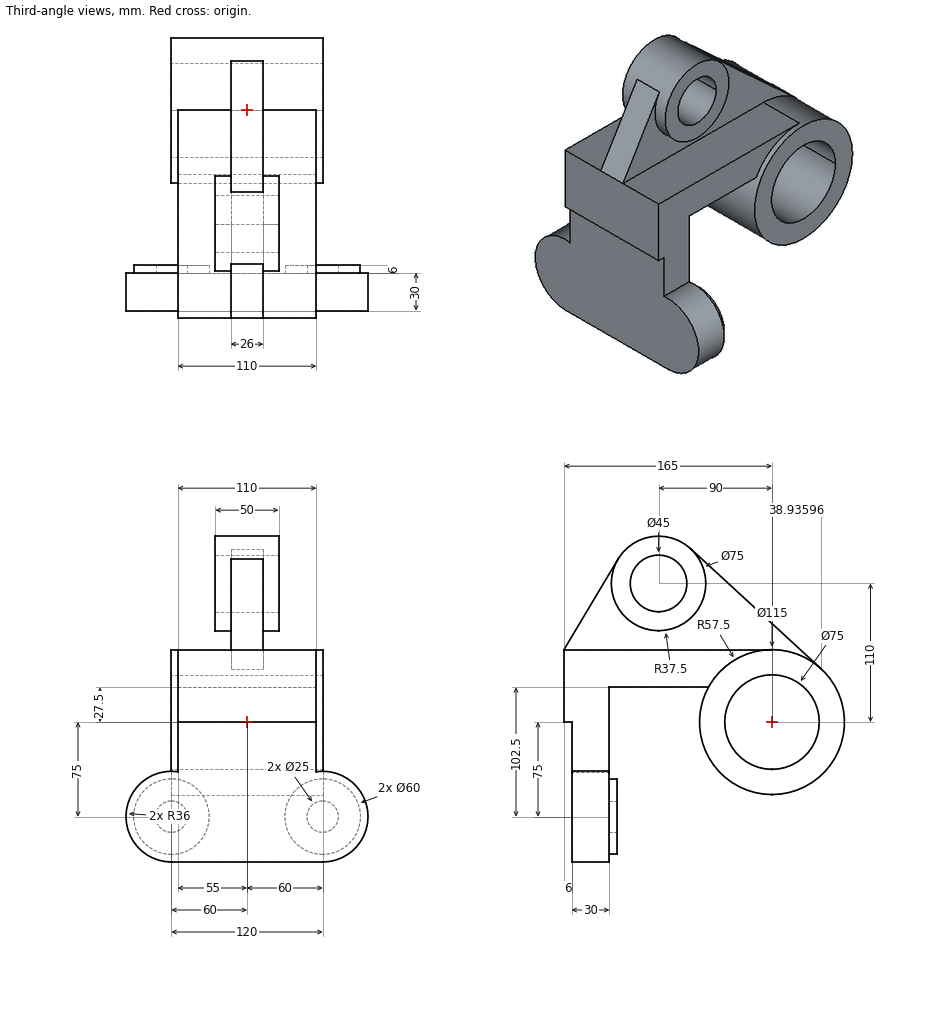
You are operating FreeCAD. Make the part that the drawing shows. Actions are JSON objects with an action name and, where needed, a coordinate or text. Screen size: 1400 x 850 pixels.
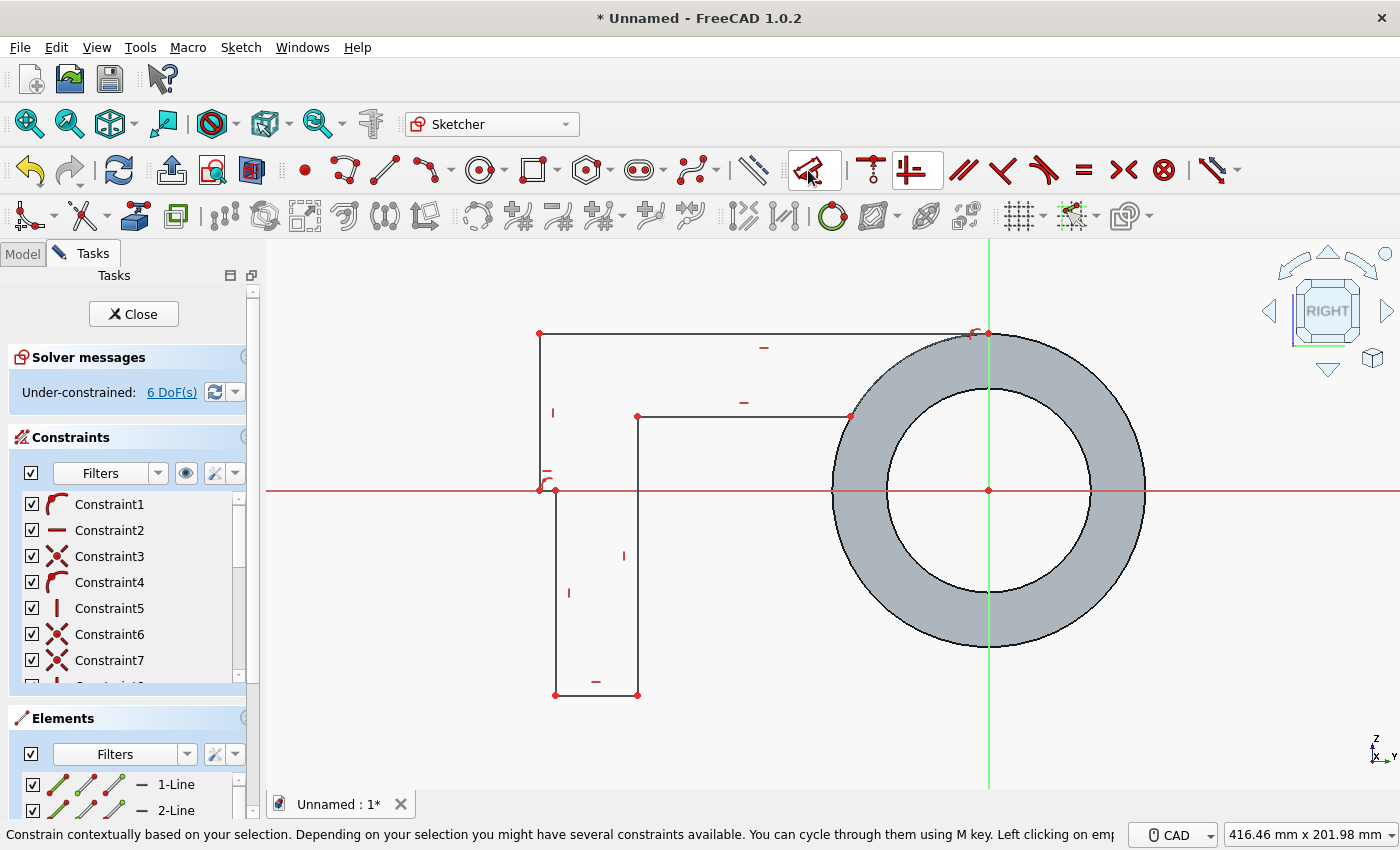
{"action": "left_click", "coordinate": [882, 376]}
{"action": "left_click", "coordinate": [860, 353]}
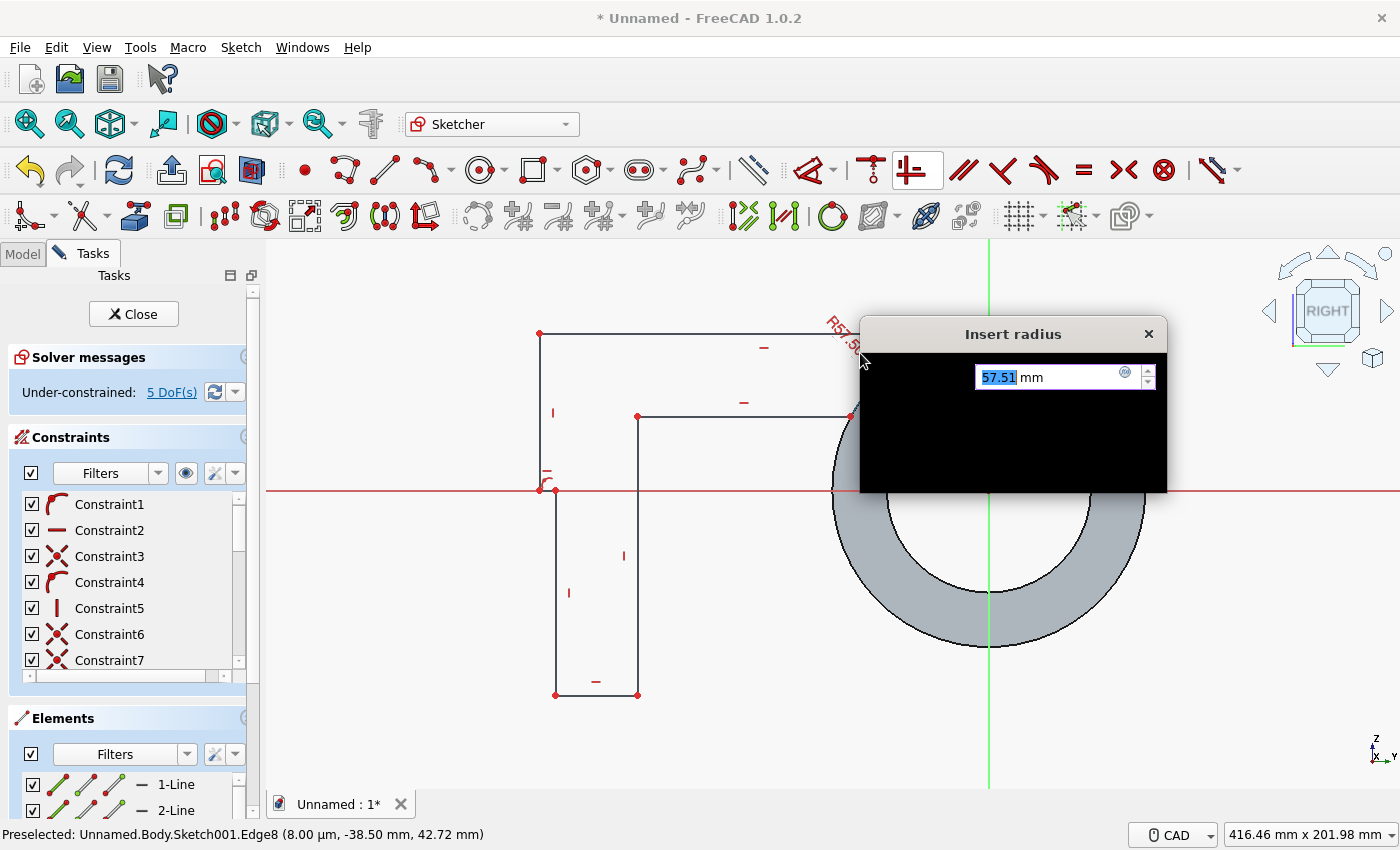
{"action": "type", "text": "57.5"}
{"action": "key", "text": "Return"}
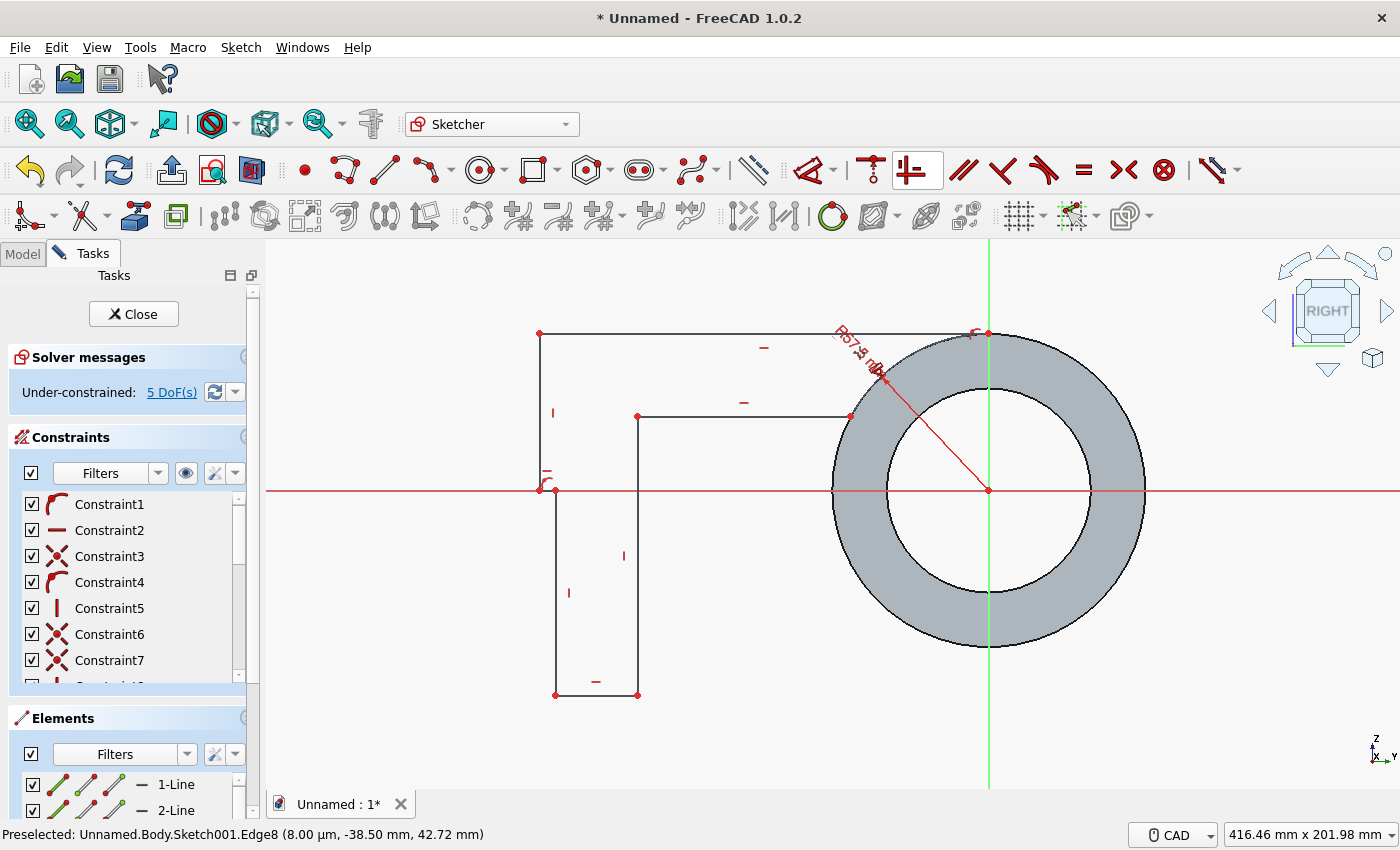
{"action": "scroll", "coordinate": [548, 490], "scroll_direction": "up", "scroll_amount": 5}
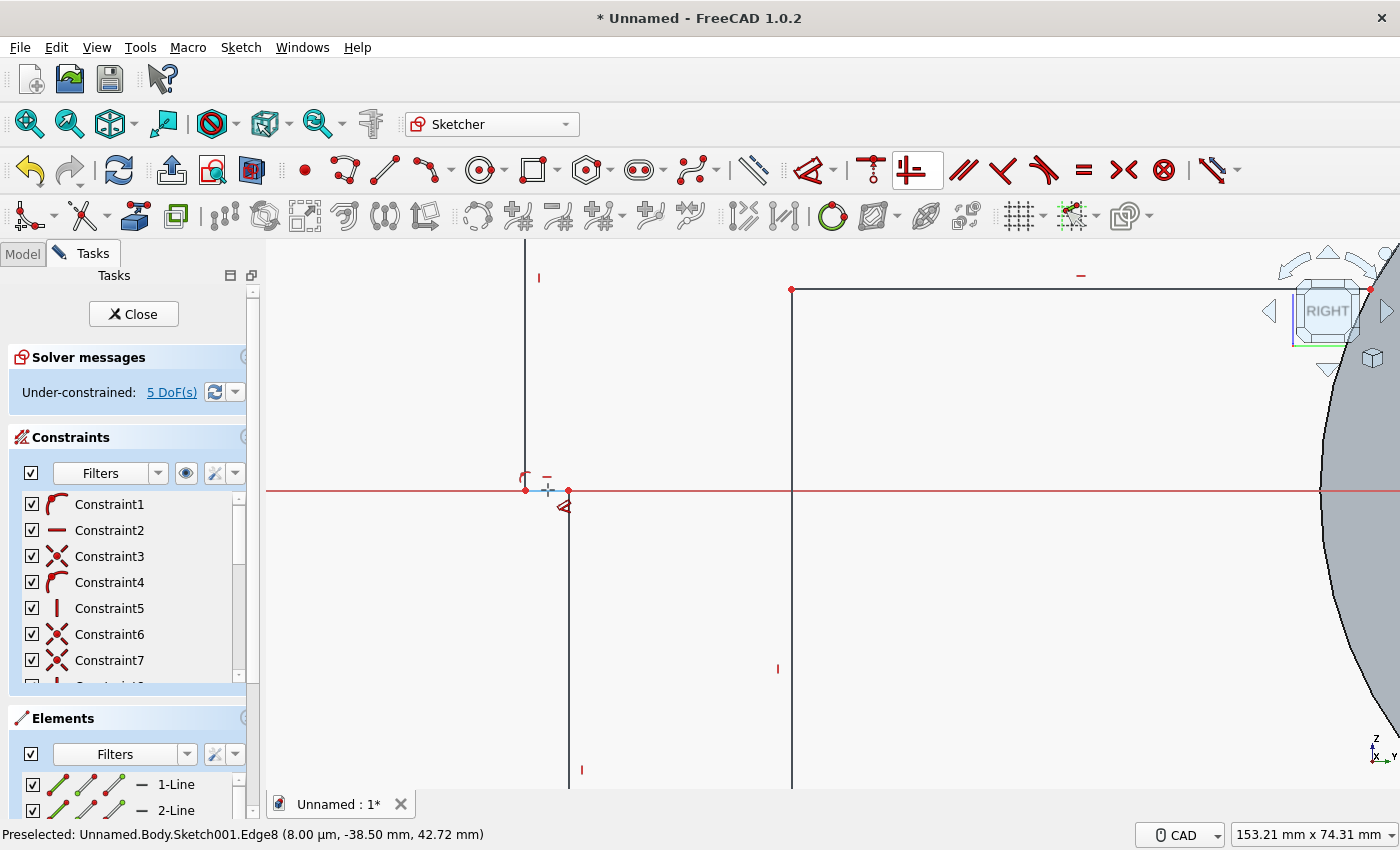
{"action": "left_click", "coordinate": [547, 491]}
{"action": "left_click", "coordinate": [547, 457]}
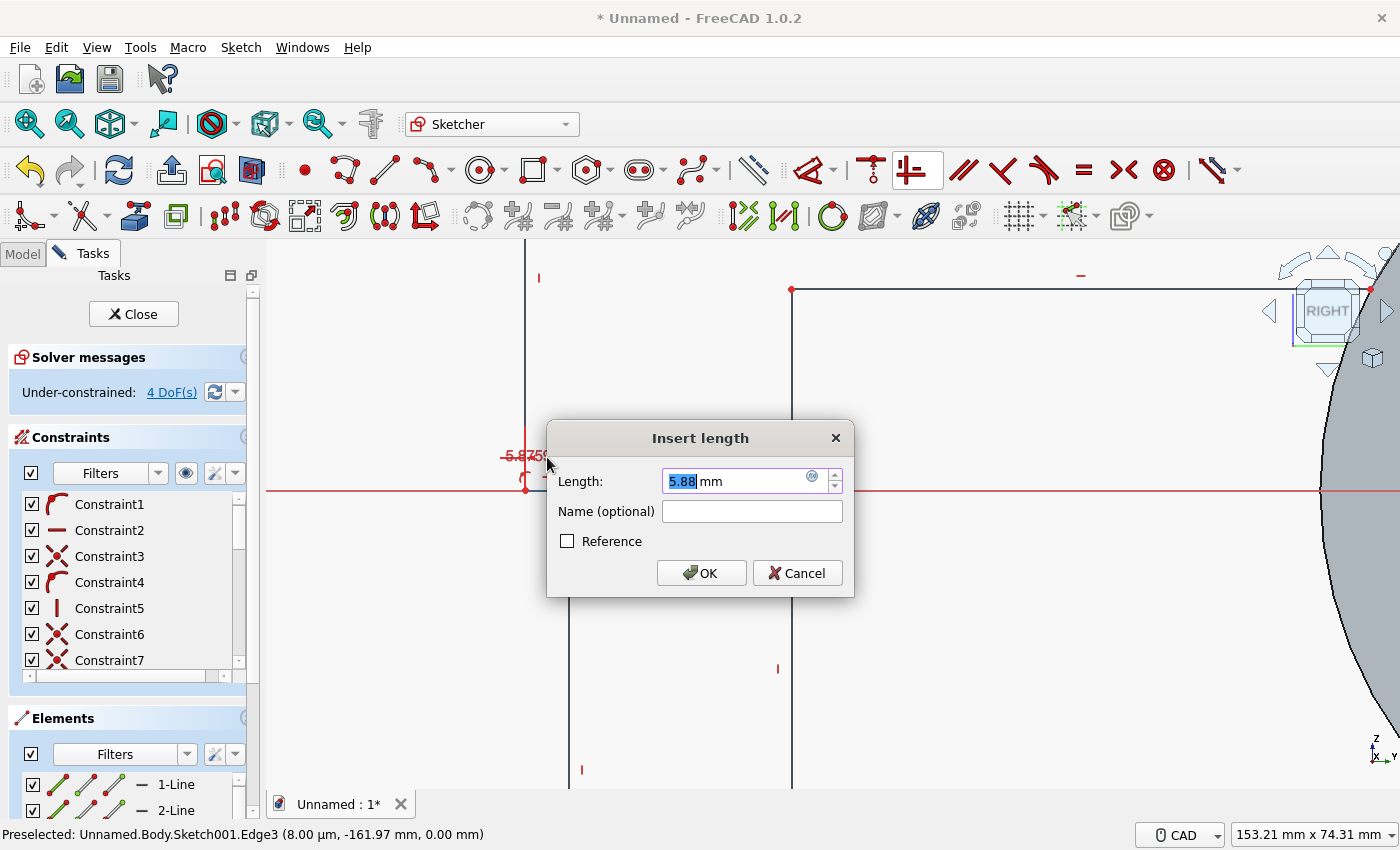
{"action": "type", "text": "6"}
{"action": "key", "text": "Return"}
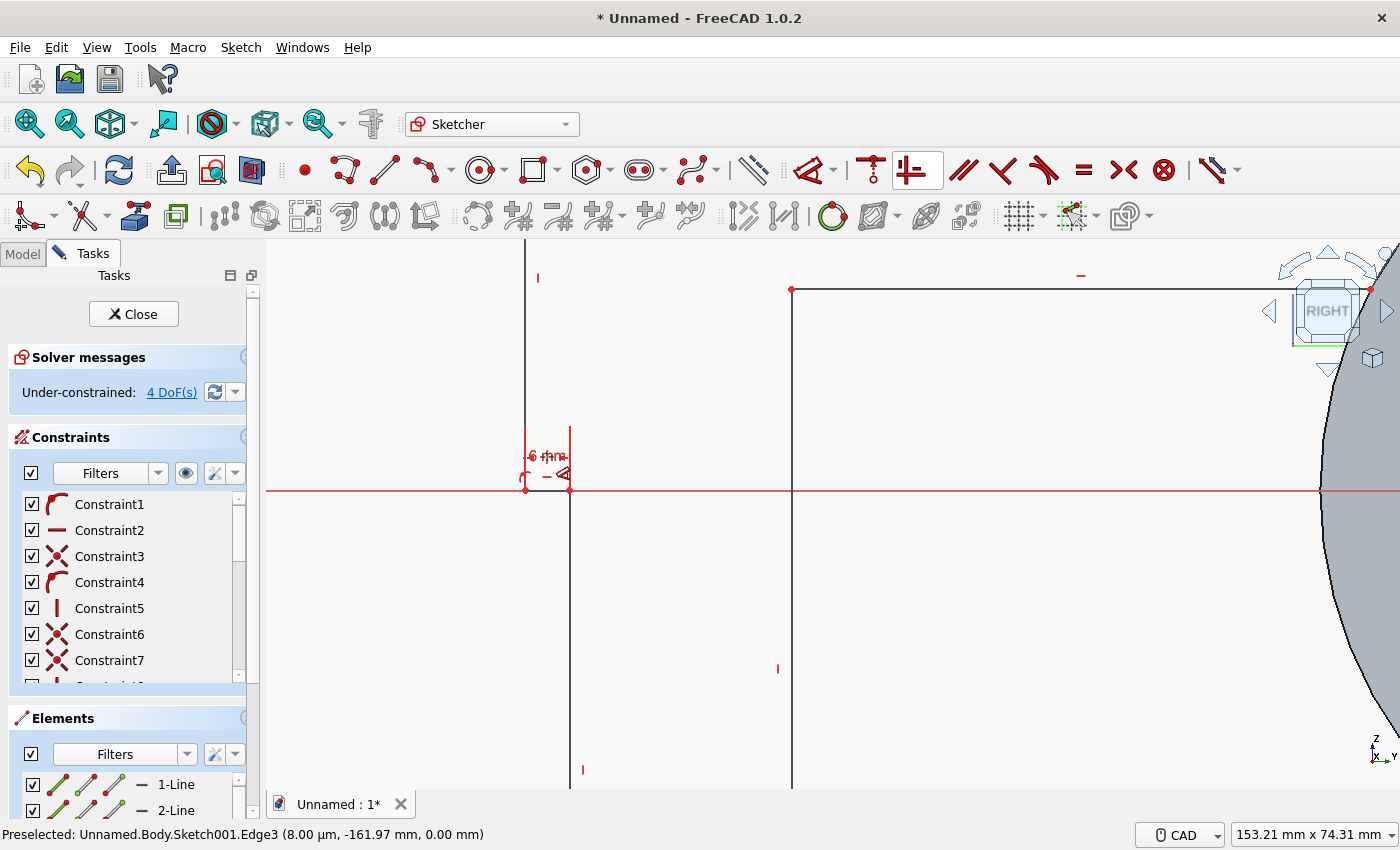
{"action": "left_click", "coordinate": [570, 658]}
{"action": "left_click", "coordinate": [536, 626]}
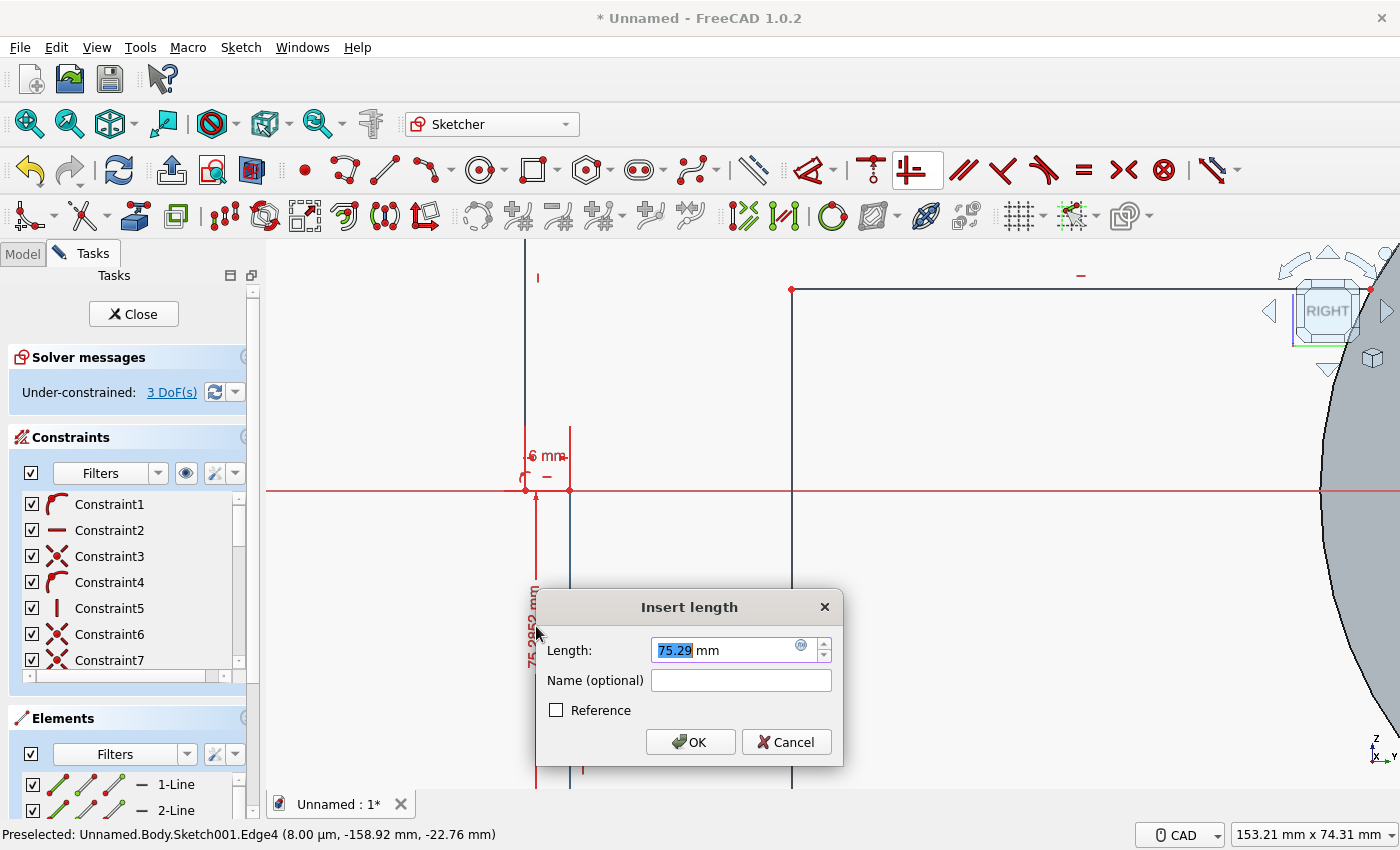
{"action": "type", "text": "75"}
{"action": "key", "text": "Return"}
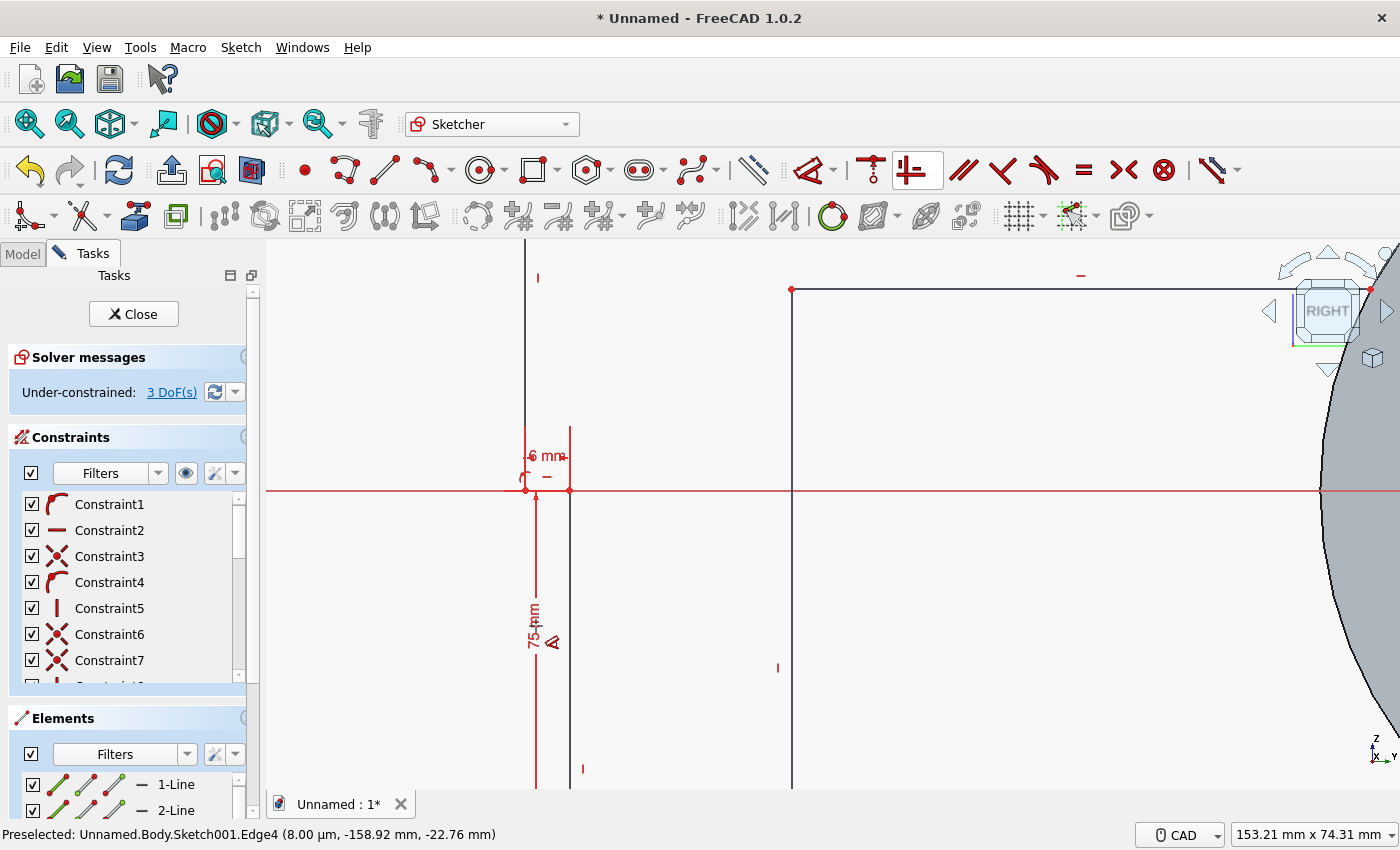
{"action": "scroll", "coordinate": [549, 490], "scroll_direction": "down", "scroll_amount": 5}